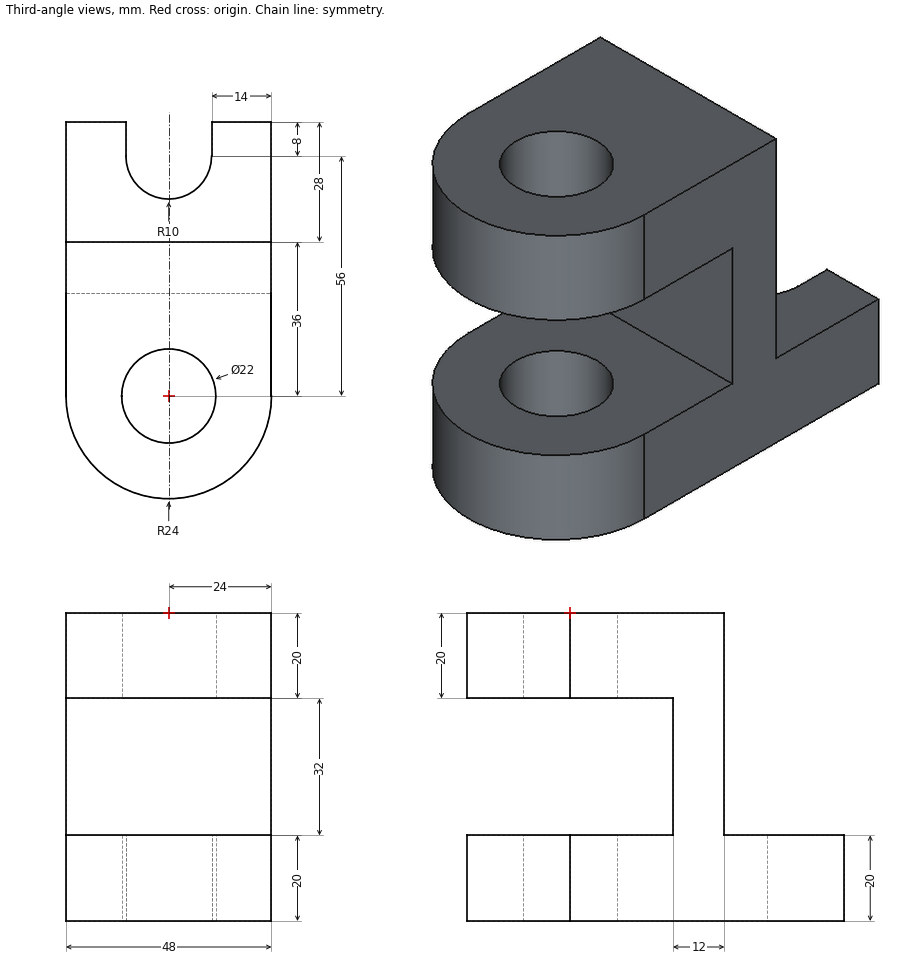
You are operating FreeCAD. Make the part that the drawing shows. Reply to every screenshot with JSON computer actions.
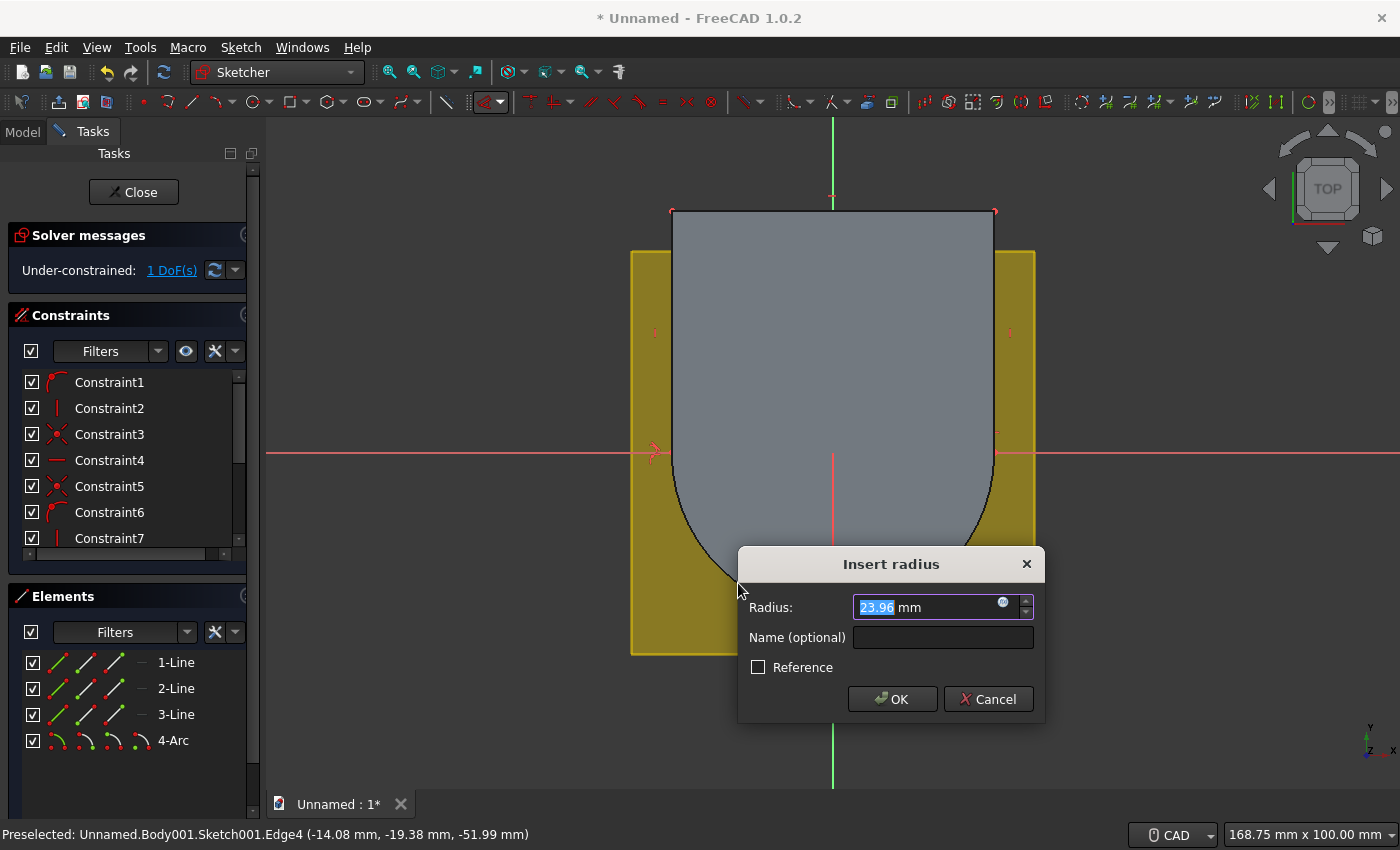
{"action": "type", "text": "24"}
{"action": "key", "text": "Return"}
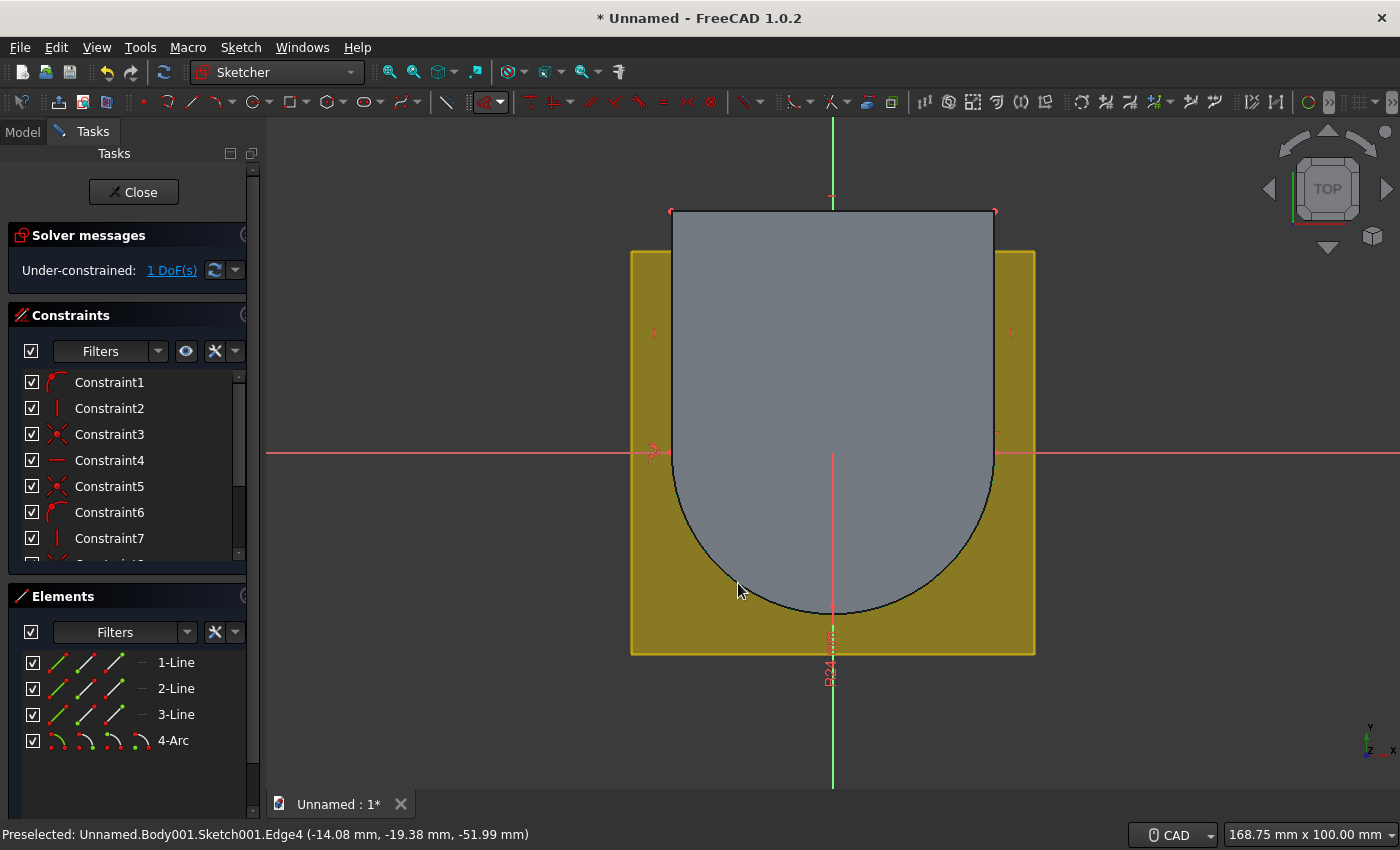
{"action": "left_click", "coordinate": [672, 381]}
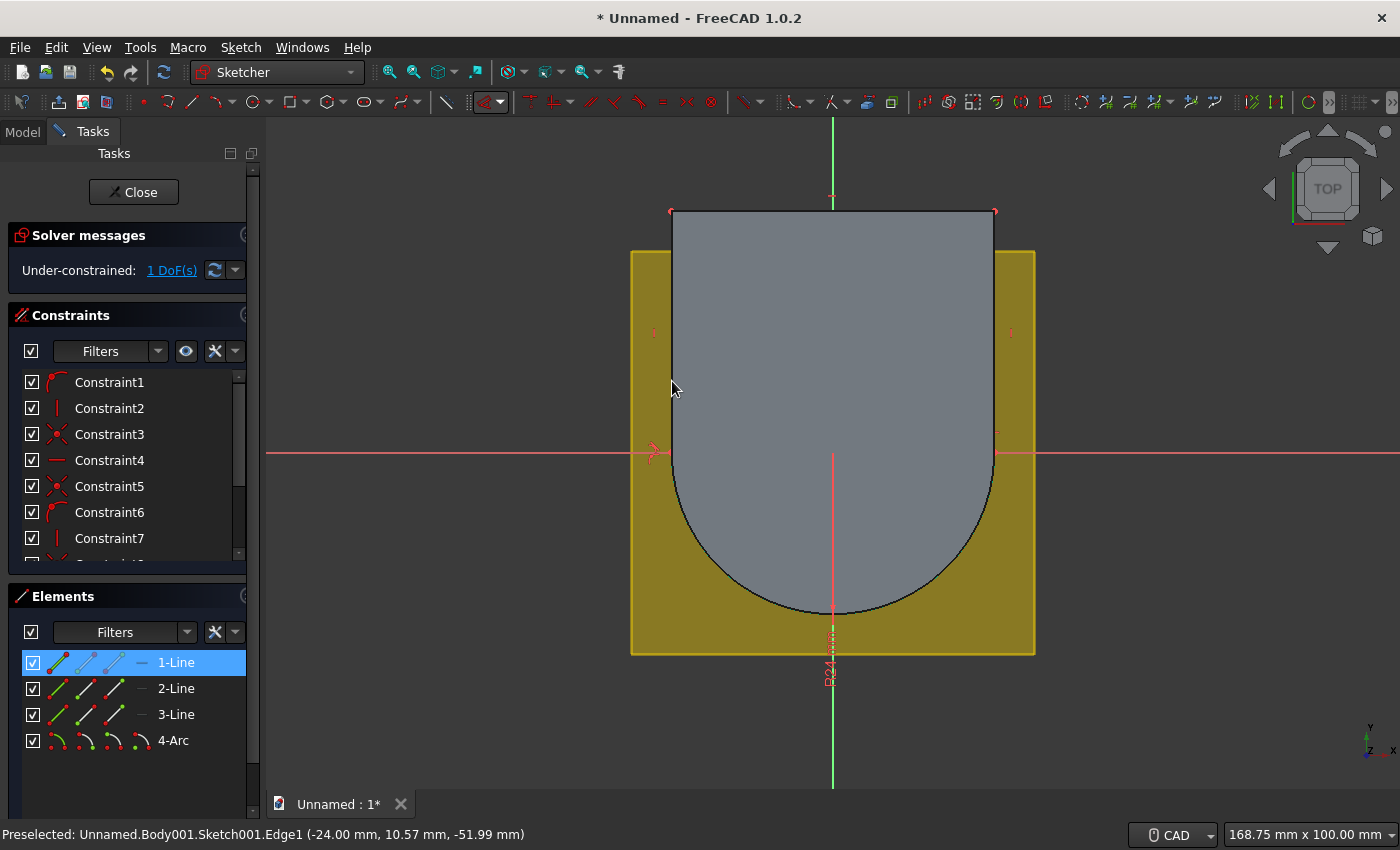
{"action": "left_click", "coordinate": [502, 102]}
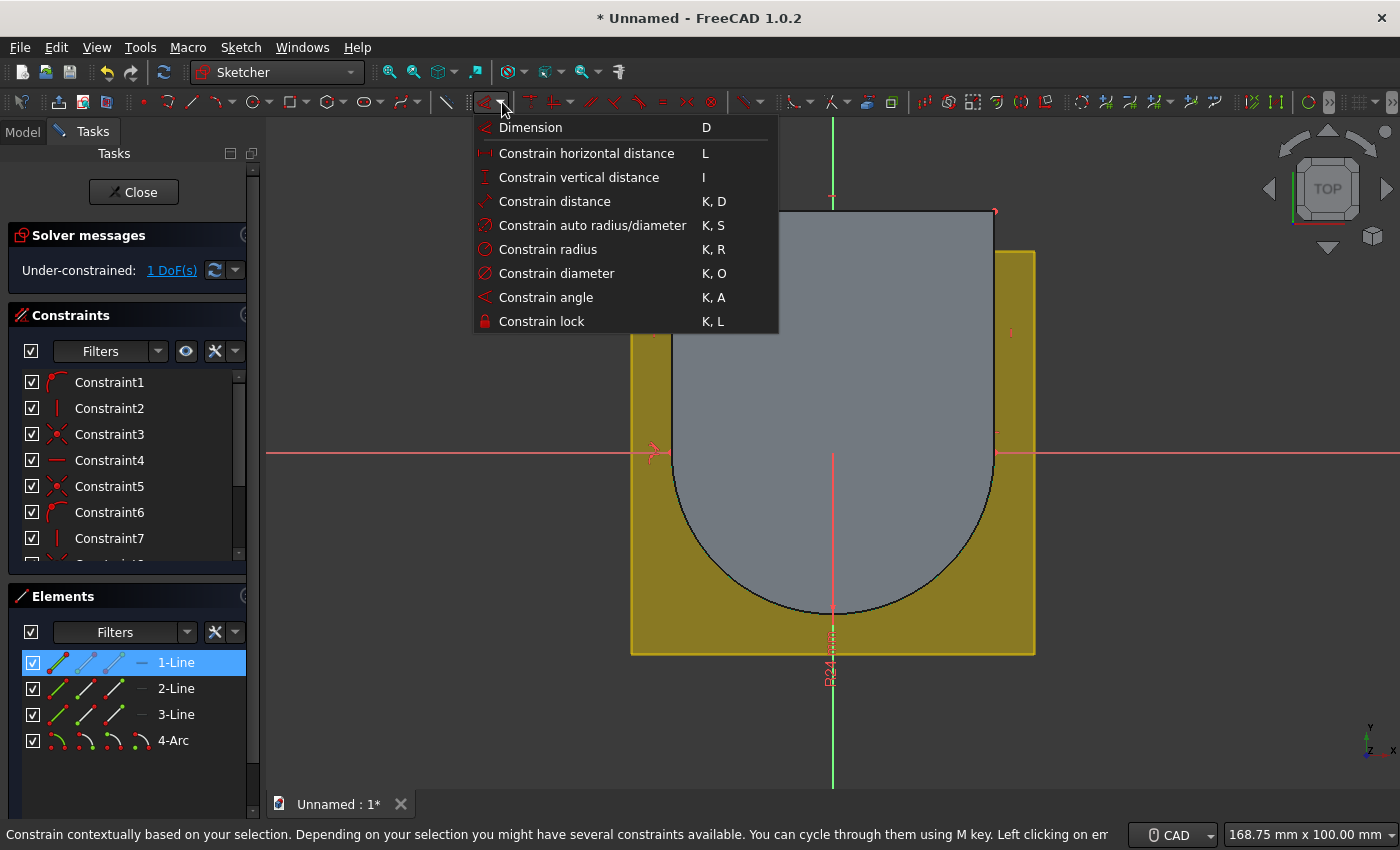
{"action": "left_click", "coordinate": [626, 177]}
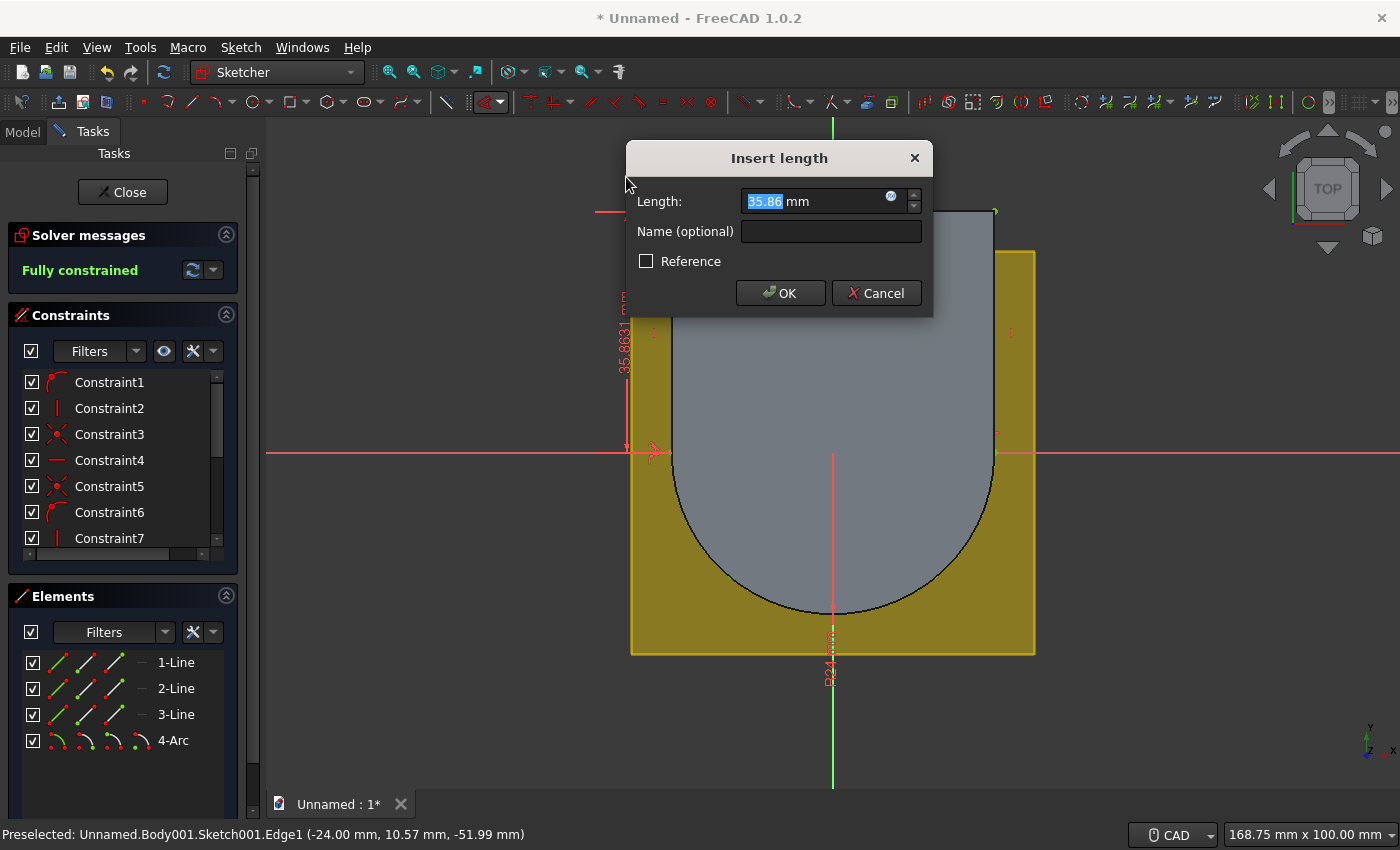
{"action": "type", "text": "36"}
{"action": "key", "text": "Return"}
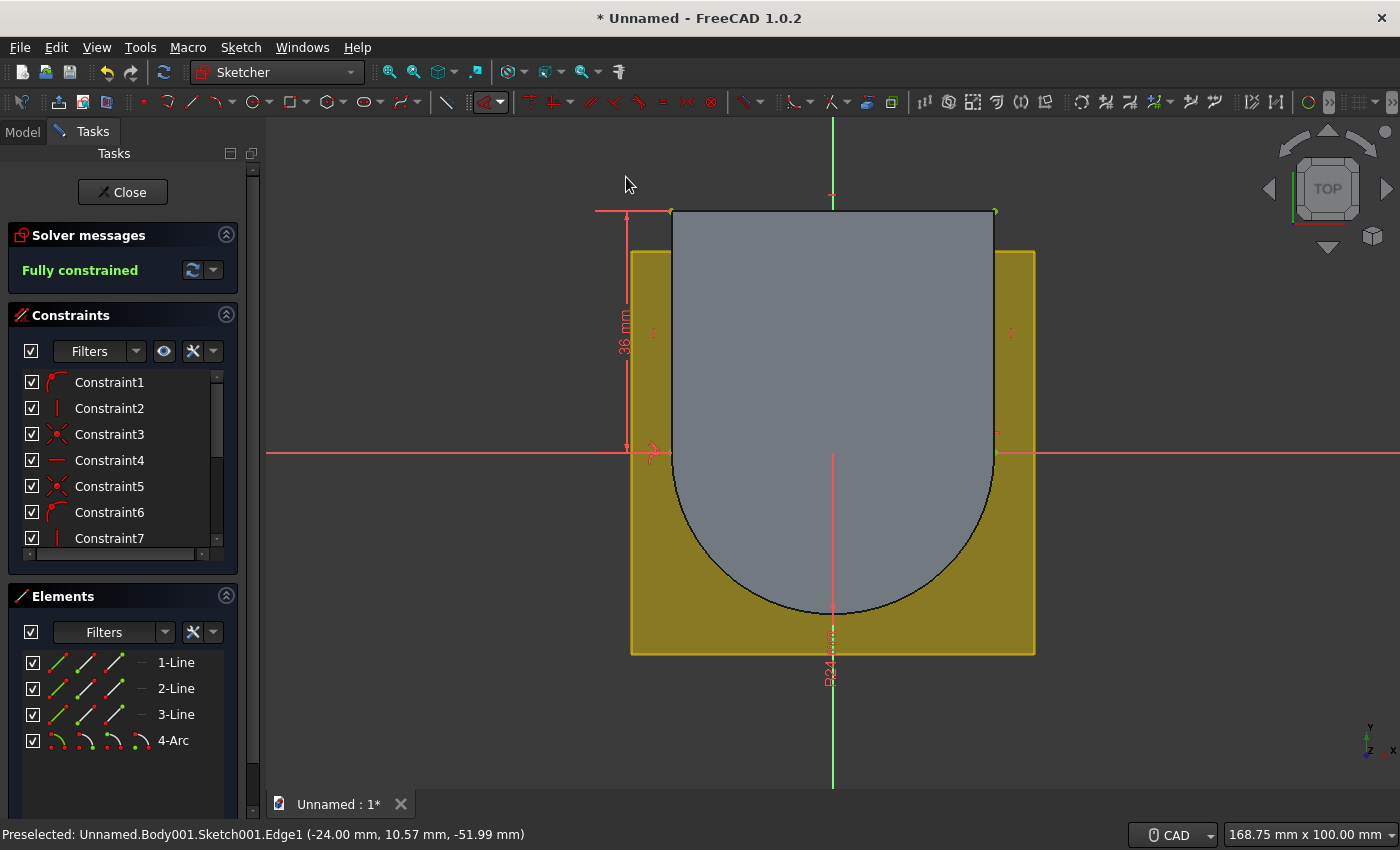
{"action": "left_click", "coordinate": [123, 192]}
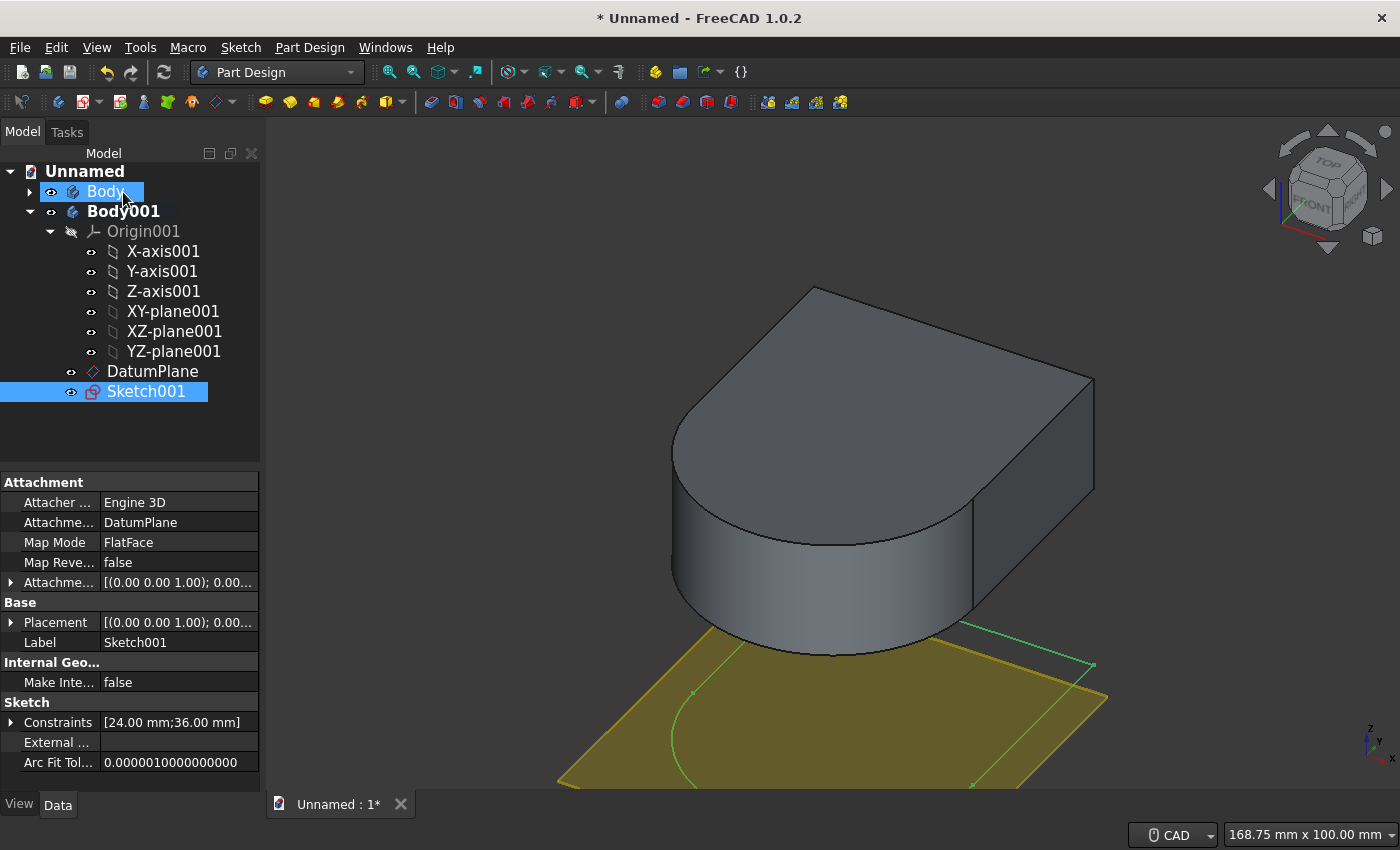
{"action": "left_click", "coordinate": [266, 102]}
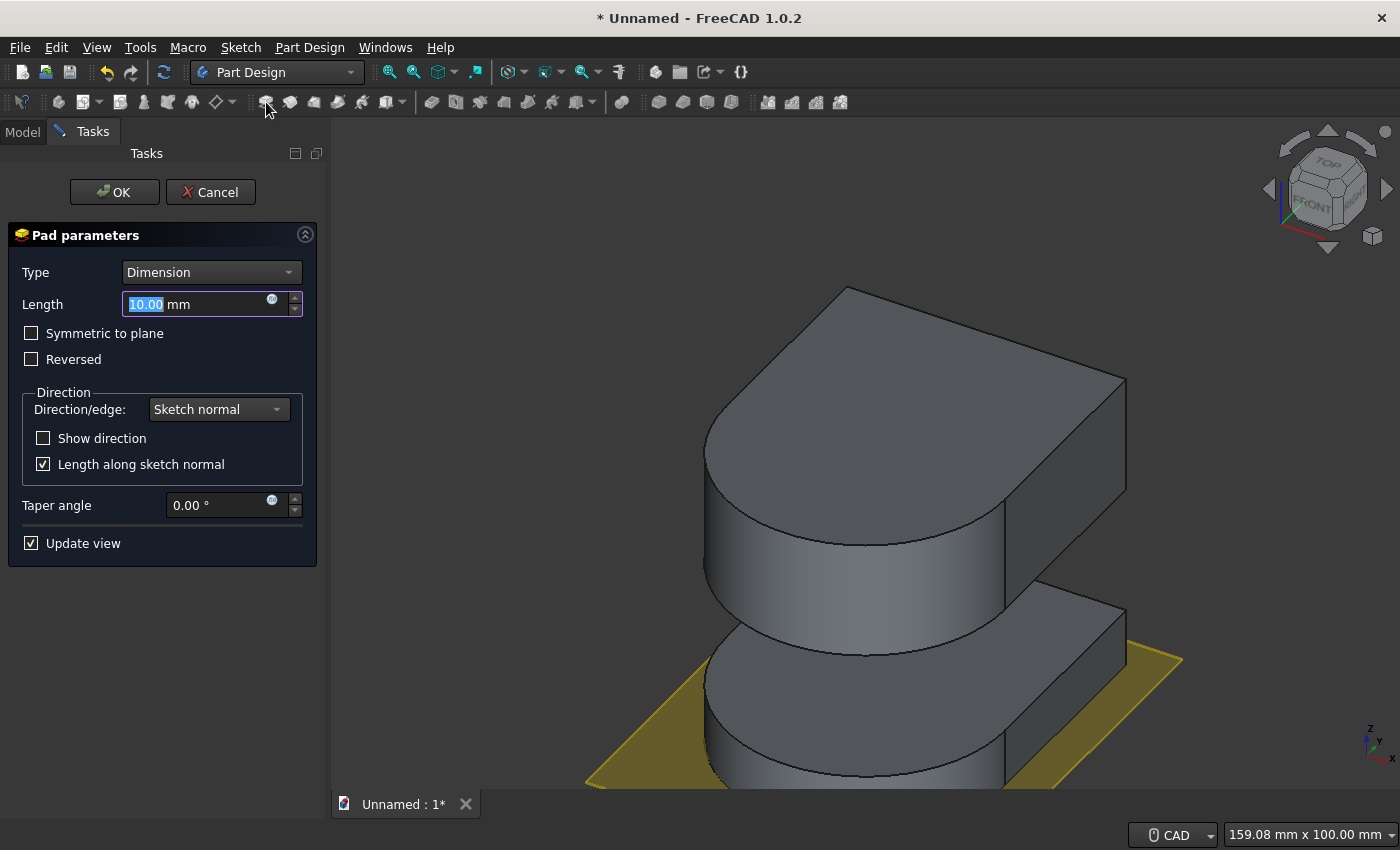
{"action": "type", "text": "20"}
{"action": "key", "text": "Tab"}